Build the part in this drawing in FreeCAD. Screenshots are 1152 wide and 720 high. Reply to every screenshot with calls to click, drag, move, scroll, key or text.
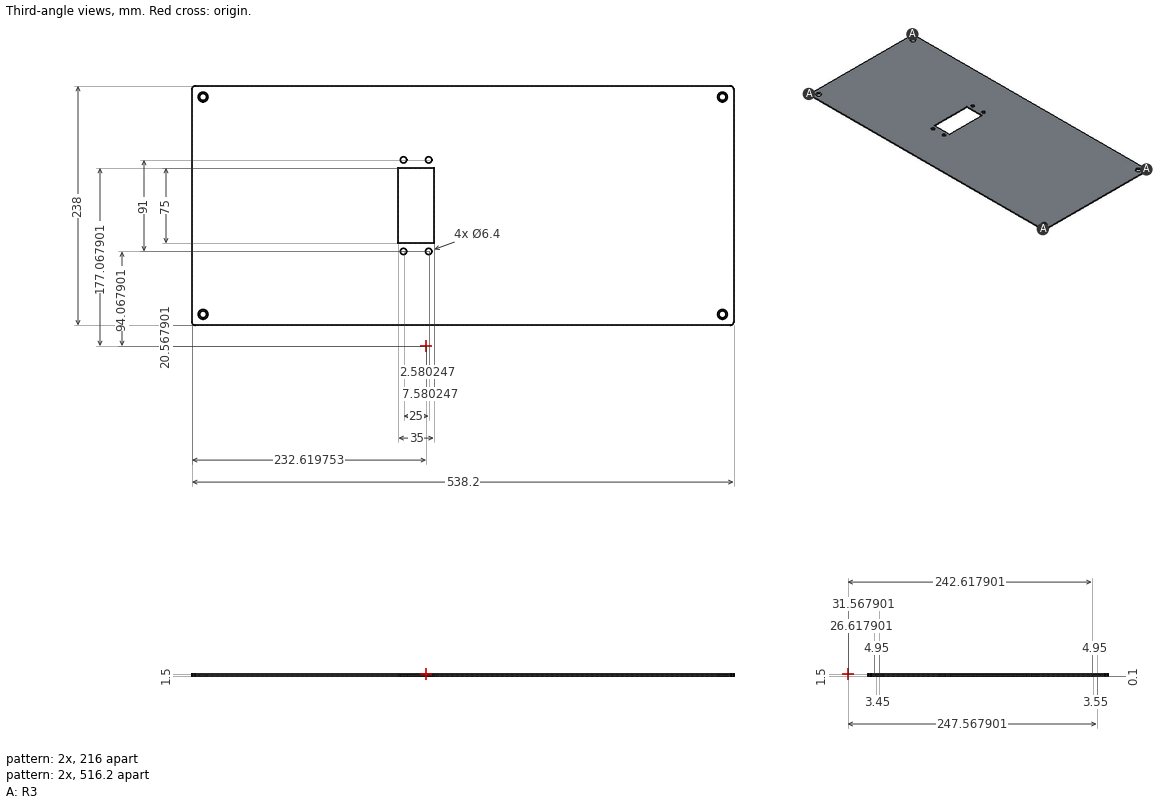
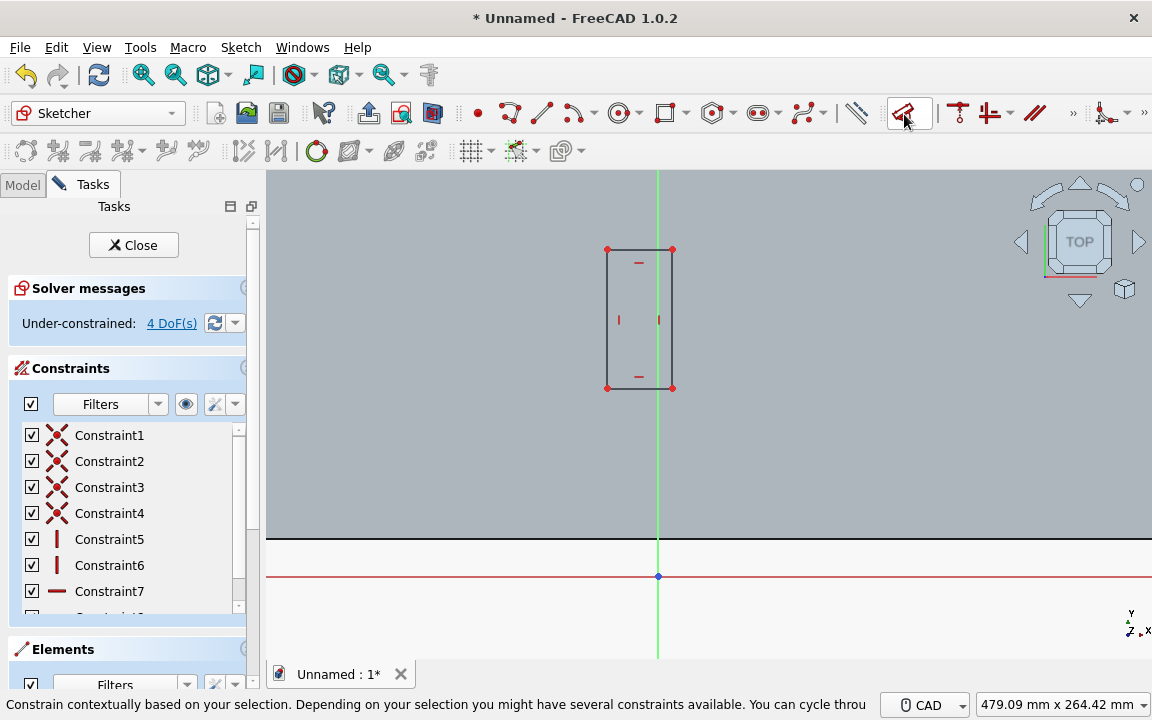
click(607, 292)
click(573, 320)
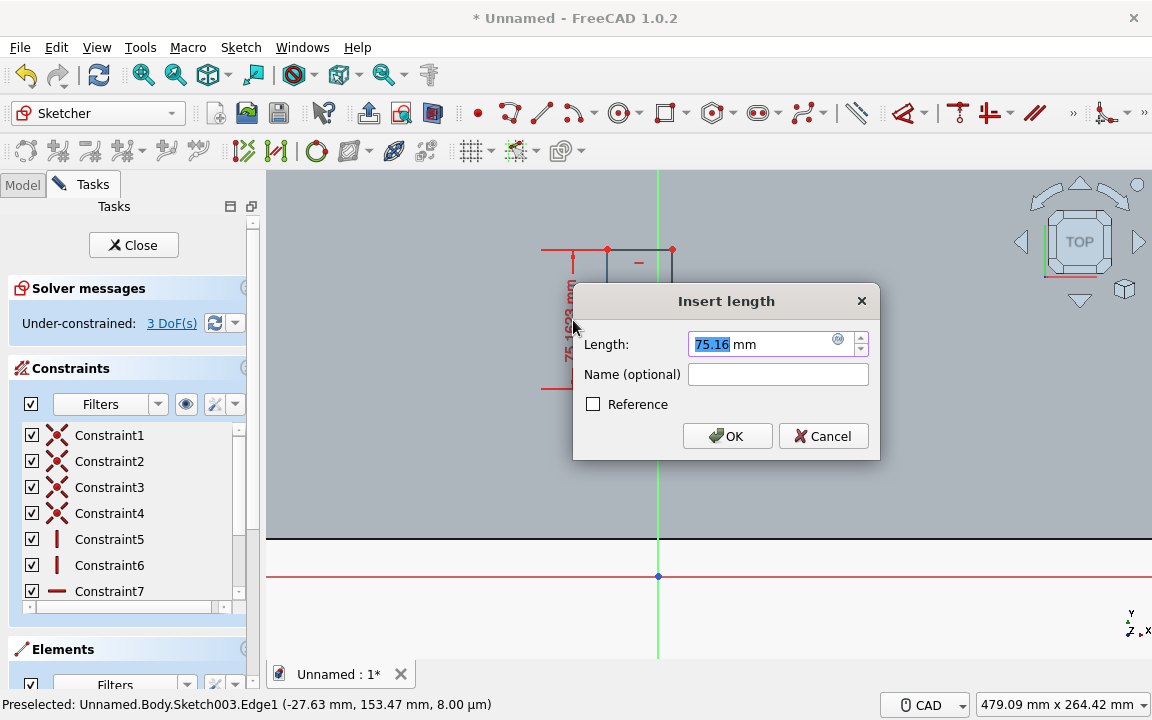
text(75)
key(Return)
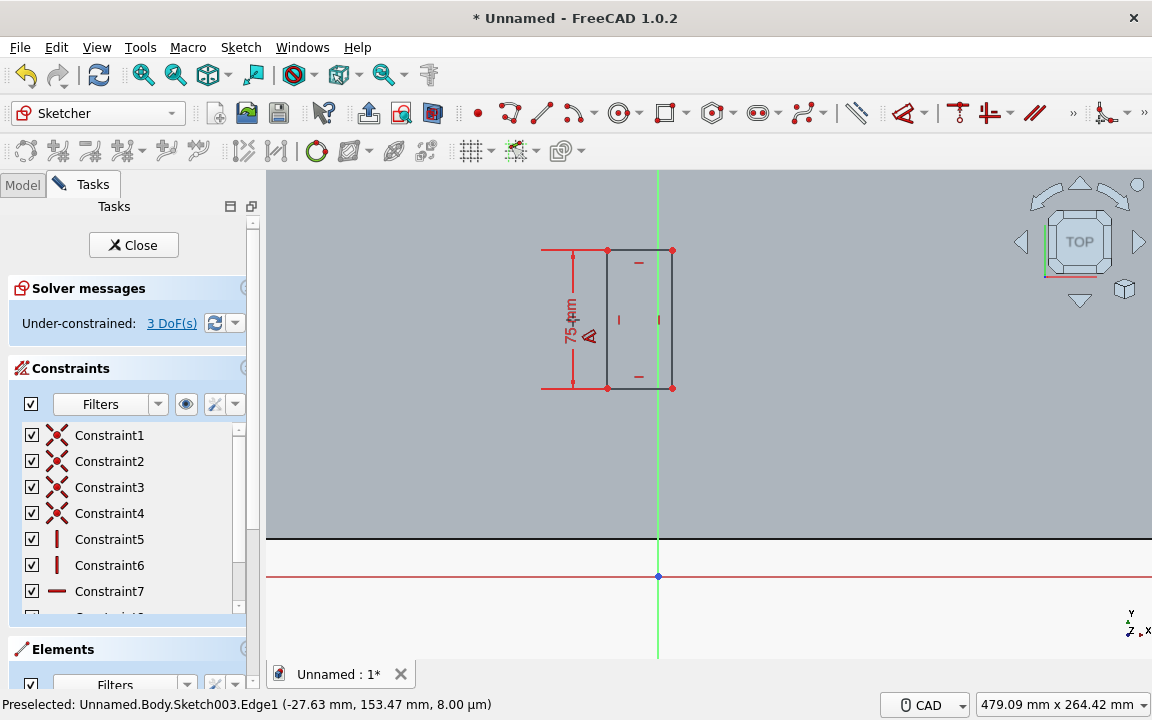
click(627, 389)
click(640, 355)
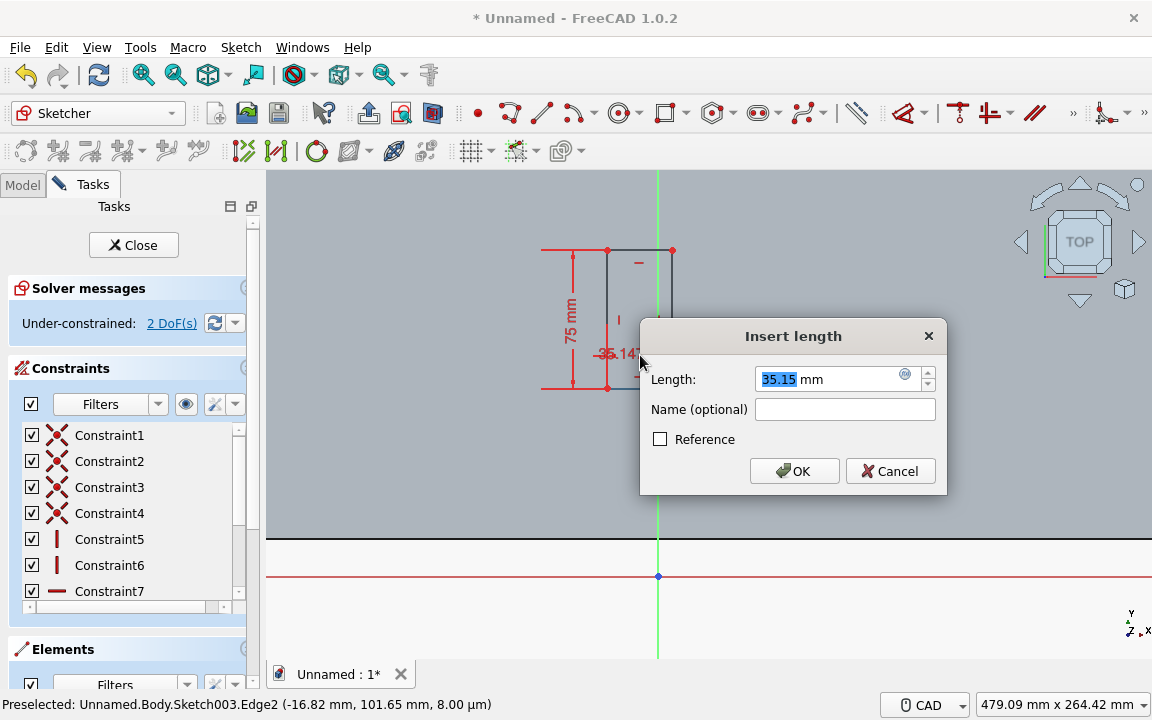
text(35)
key(Return)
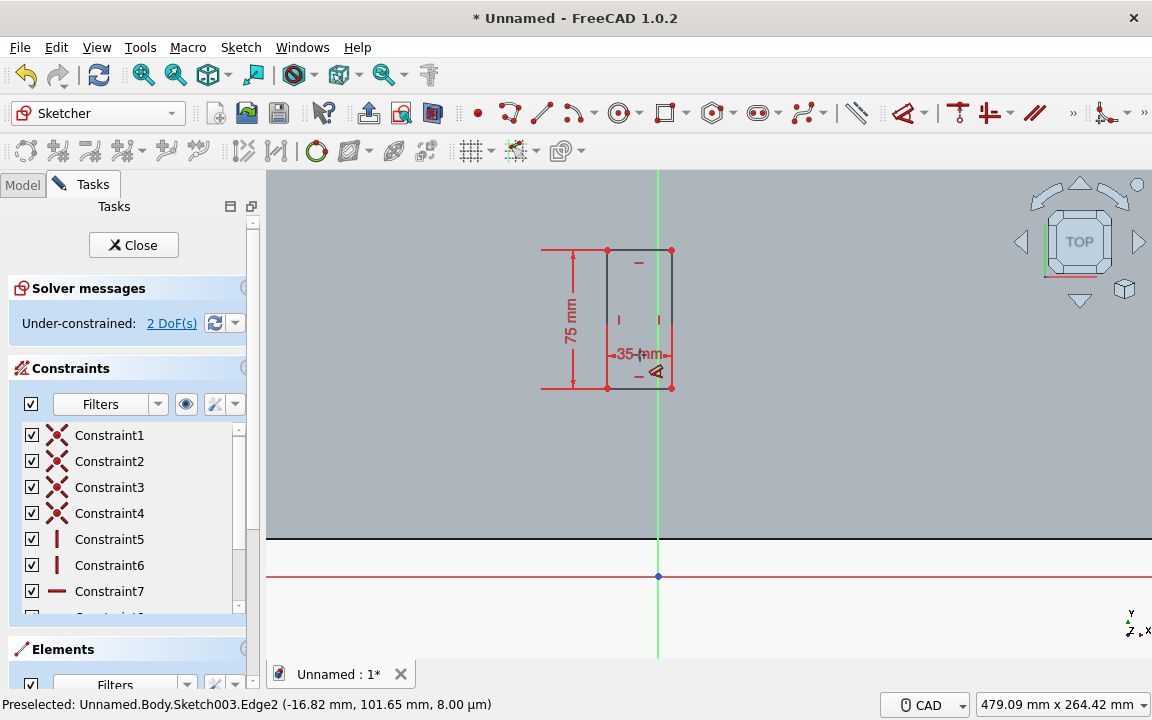
scroll(672, 389, up, 6)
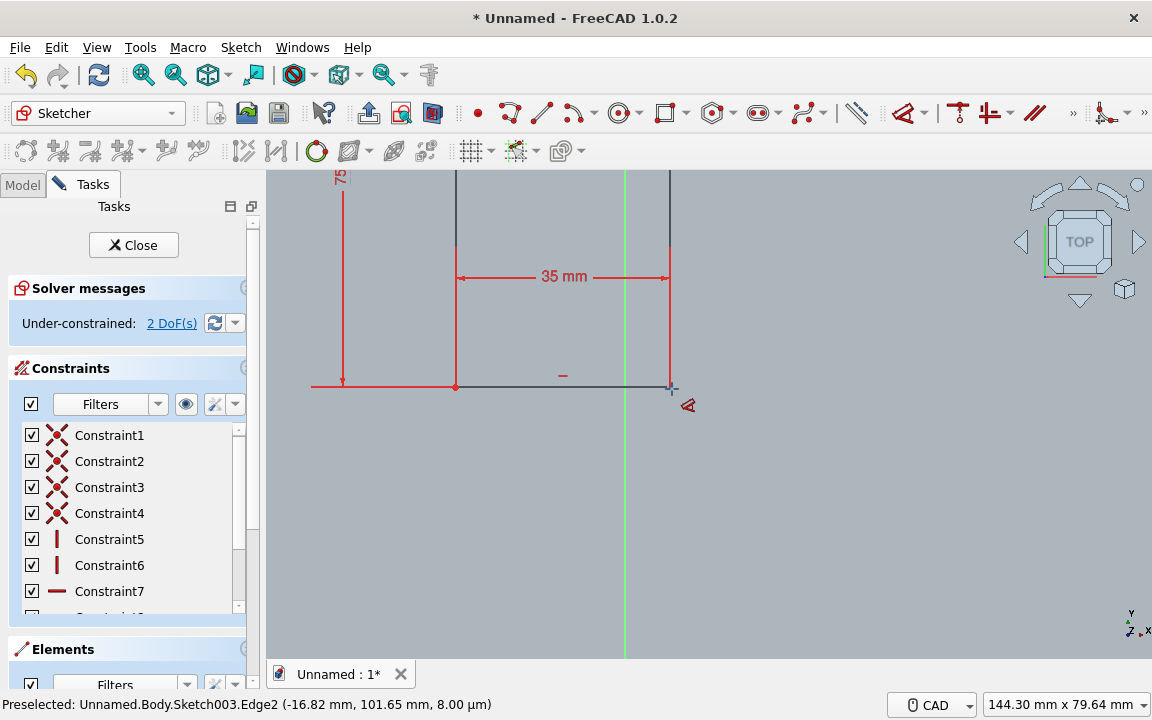
click(670, 387)
click(648, 353)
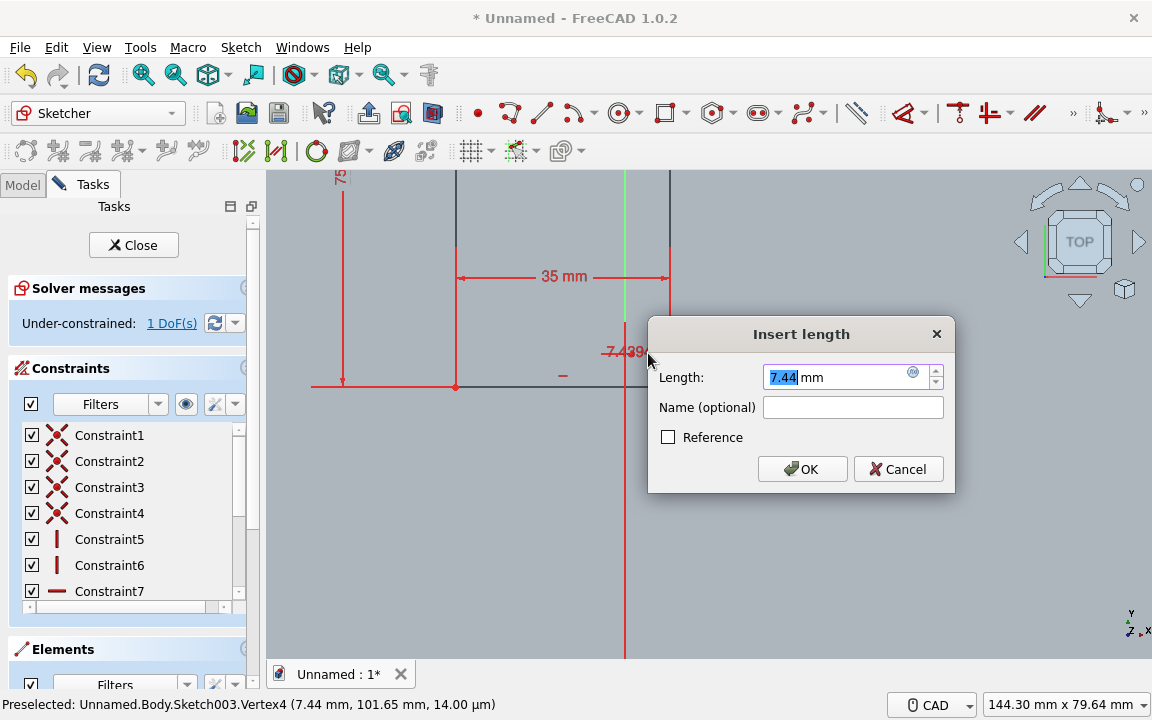
text(7.580247)
key(Return)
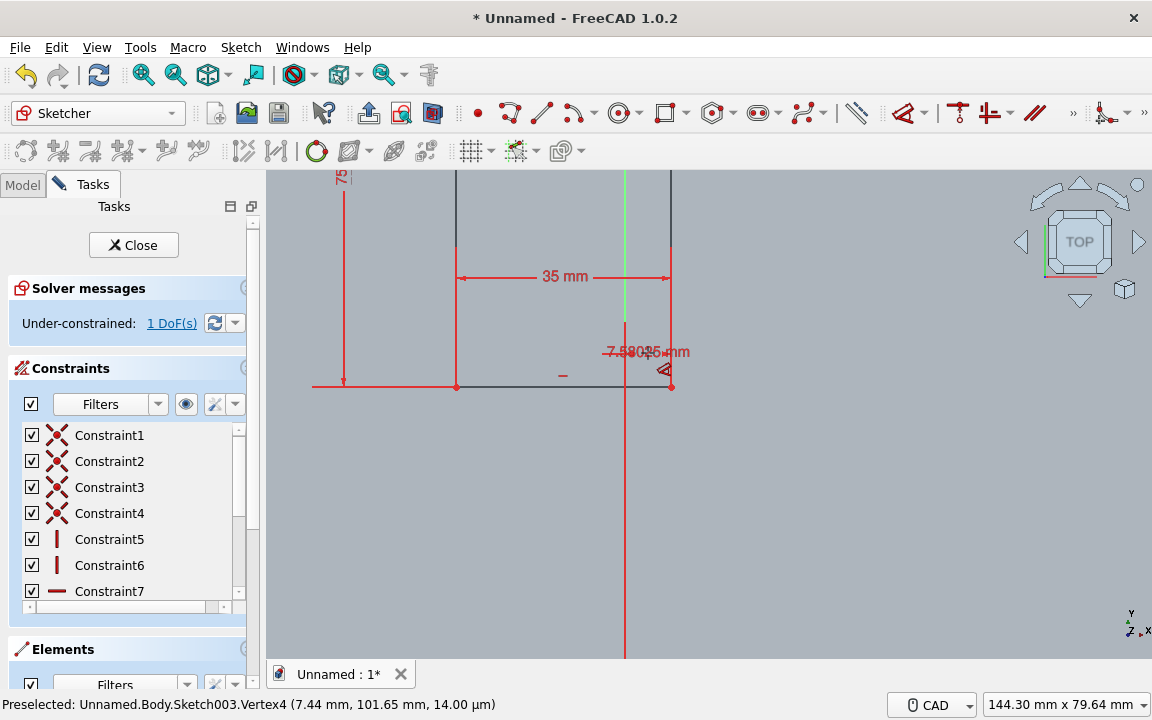
scroll(674, 391, down, 6)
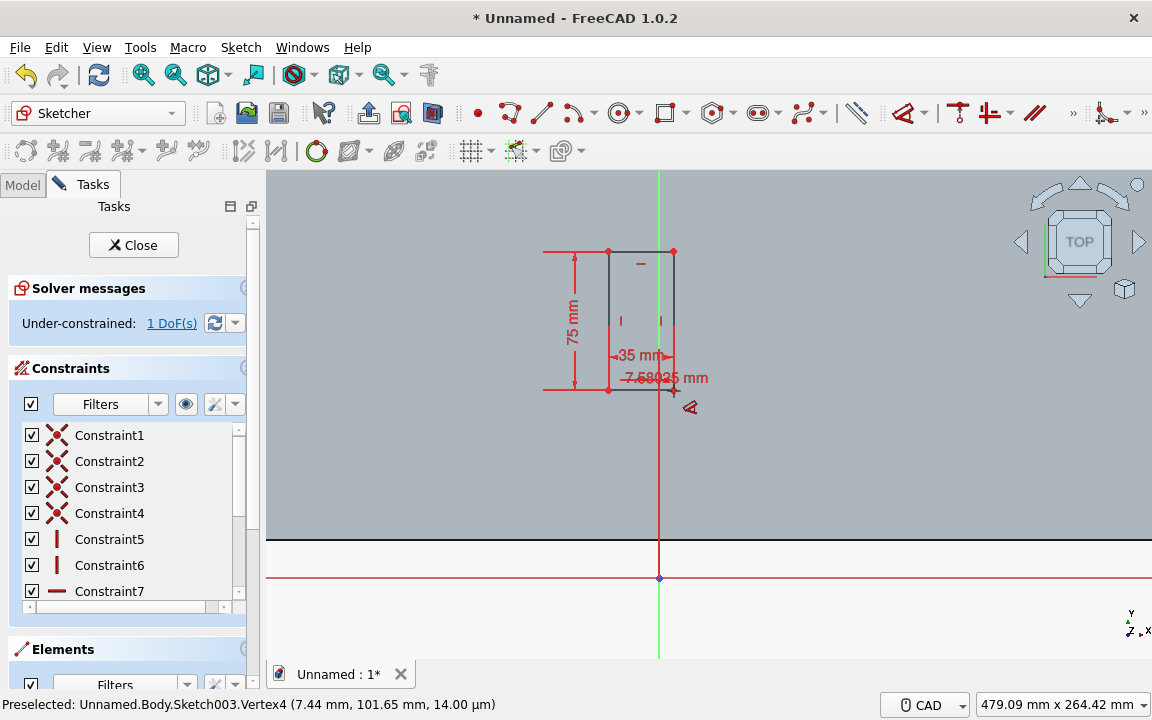
click(609, 252)
click(575, 415)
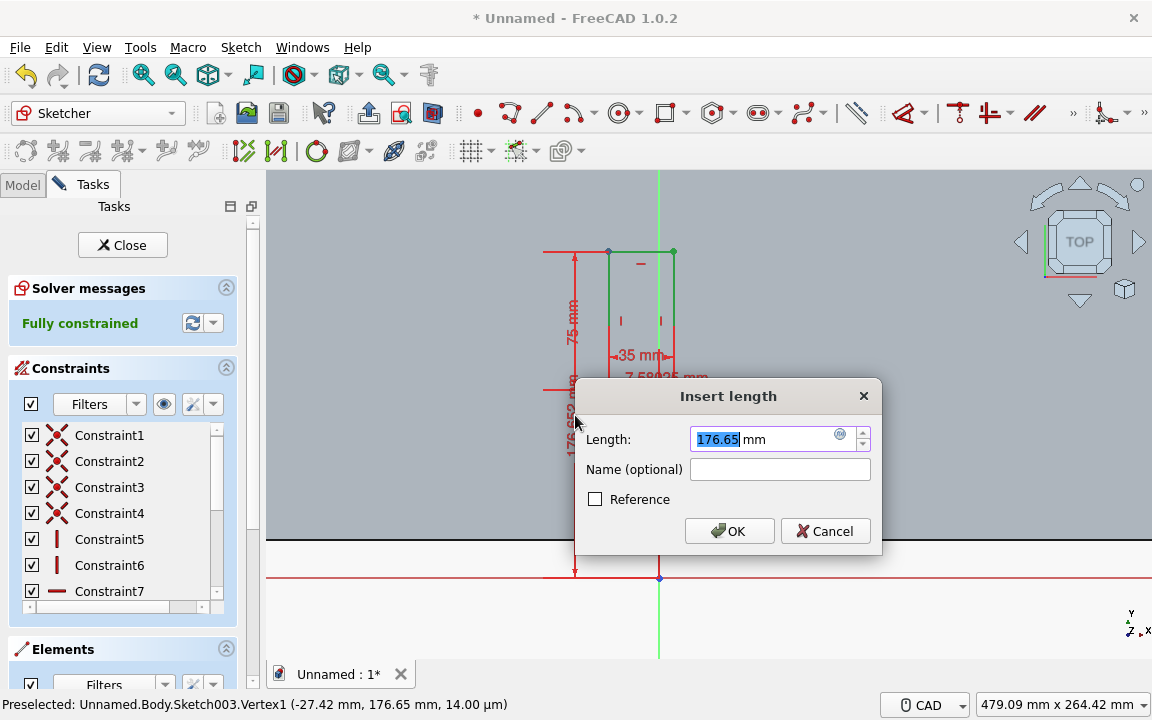
text(177.067901)
key(Return)
key(Escape)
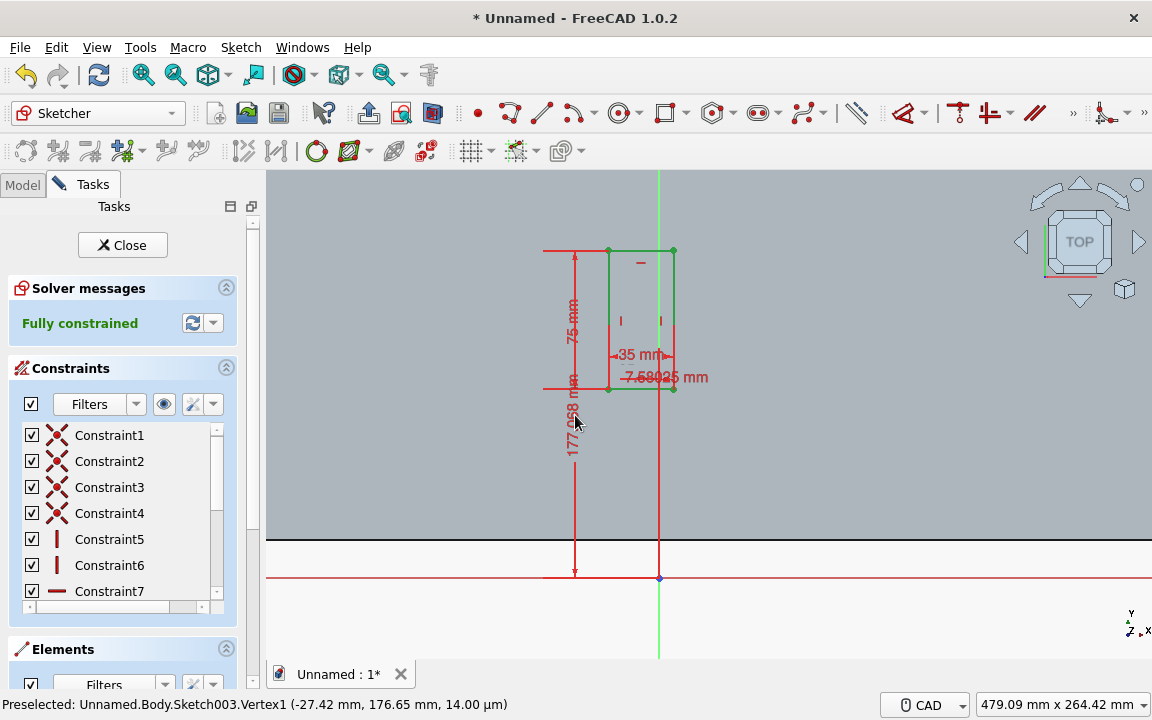
click(123, 245)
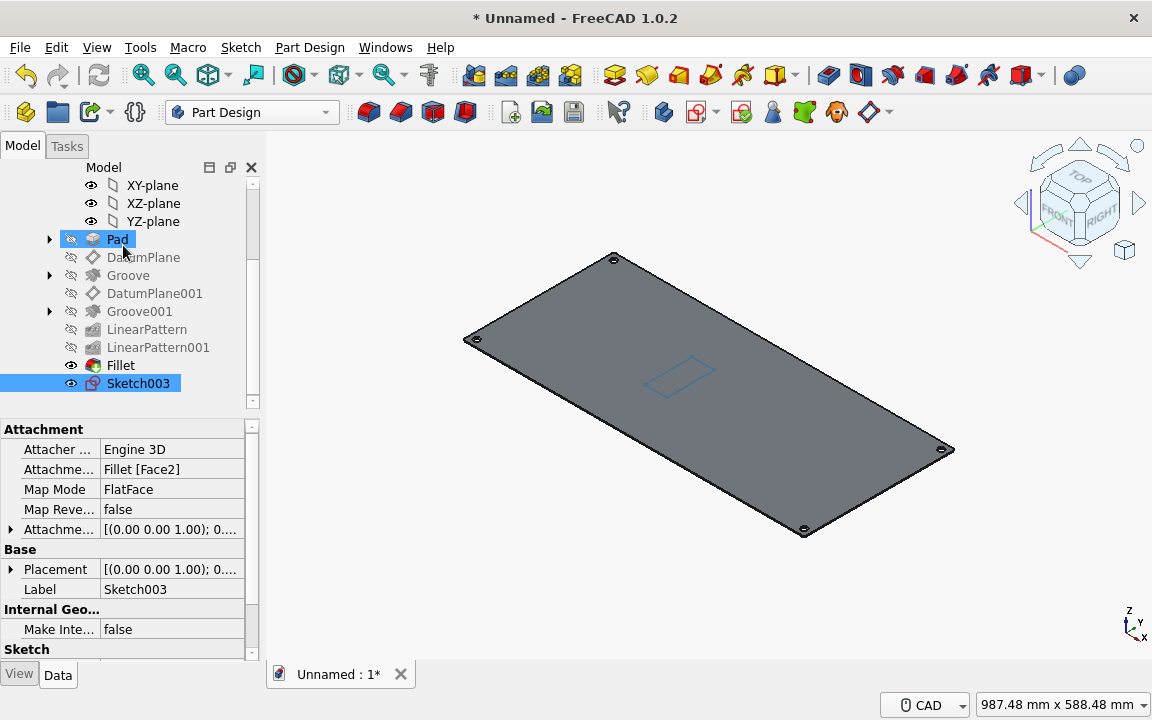
click(830, 76)